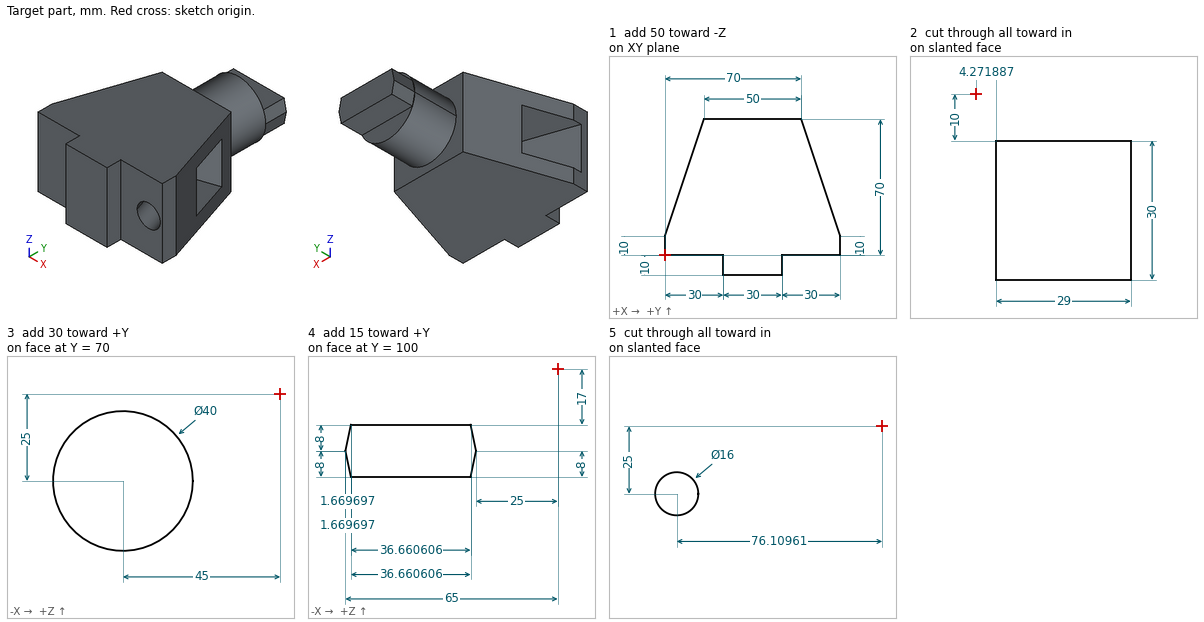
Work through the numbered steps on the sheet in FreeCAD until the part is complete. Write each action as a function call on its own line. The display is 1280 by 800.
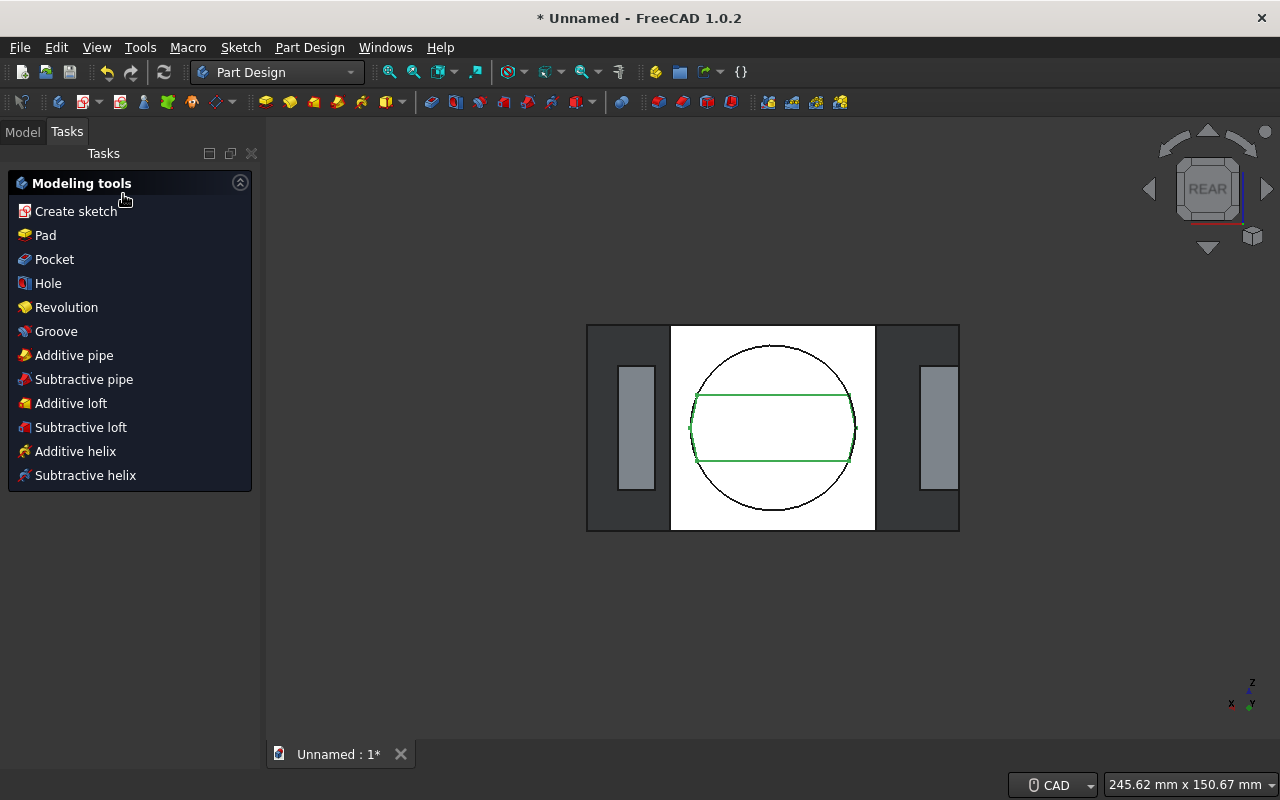
click(266, 102)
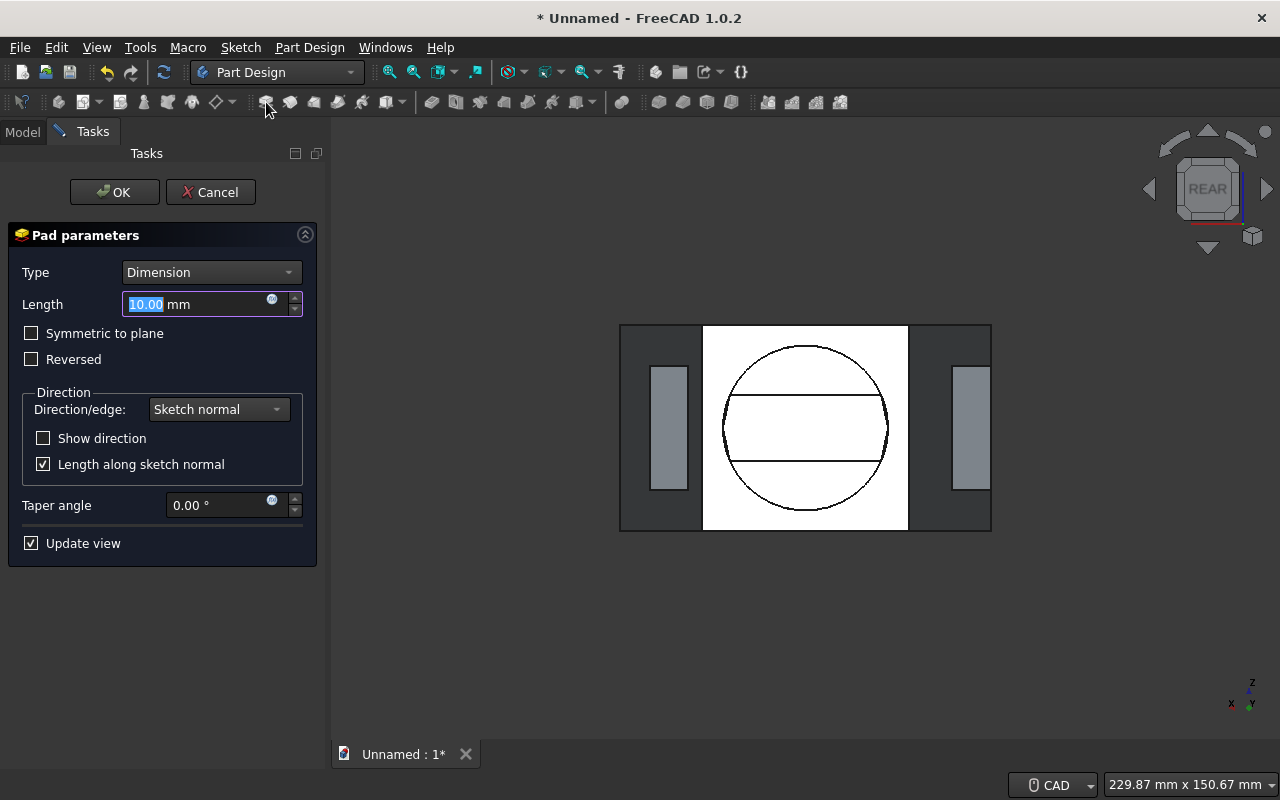
text(15)
key(Tab)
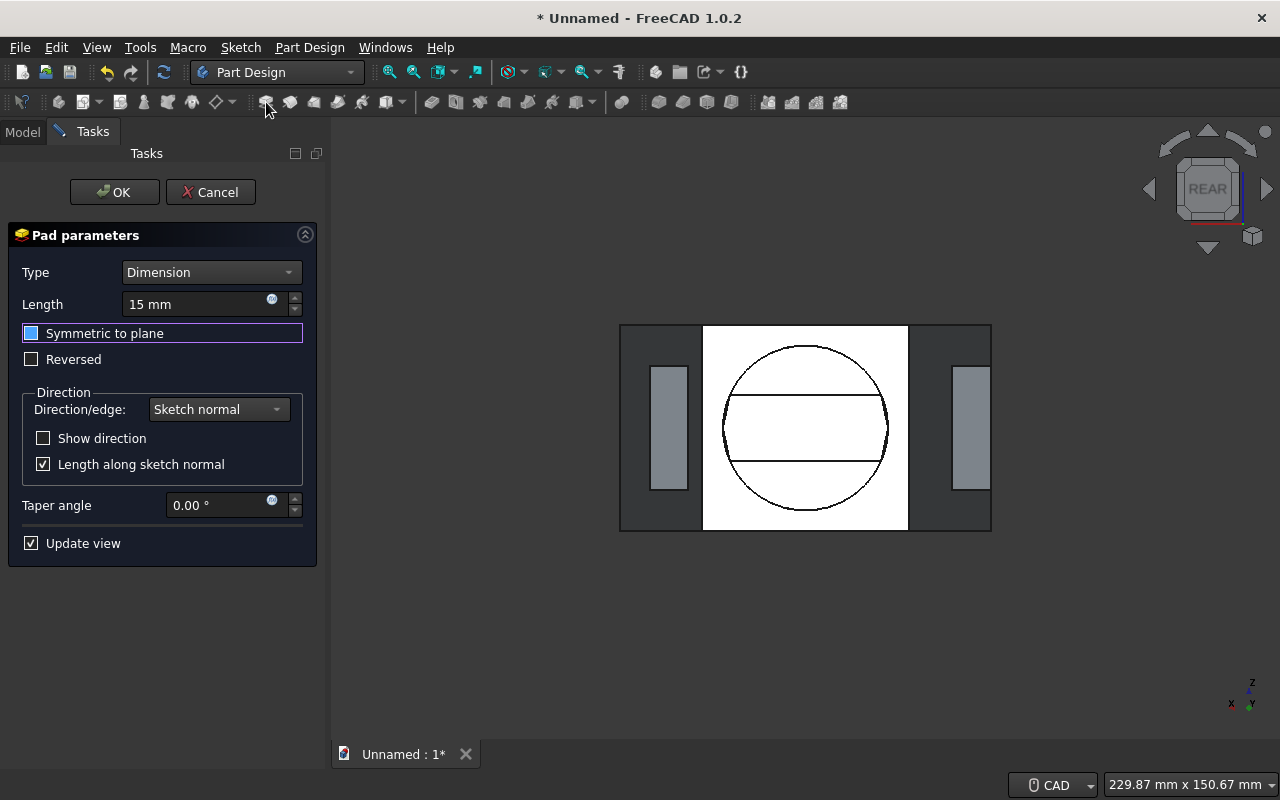
click(115, 192)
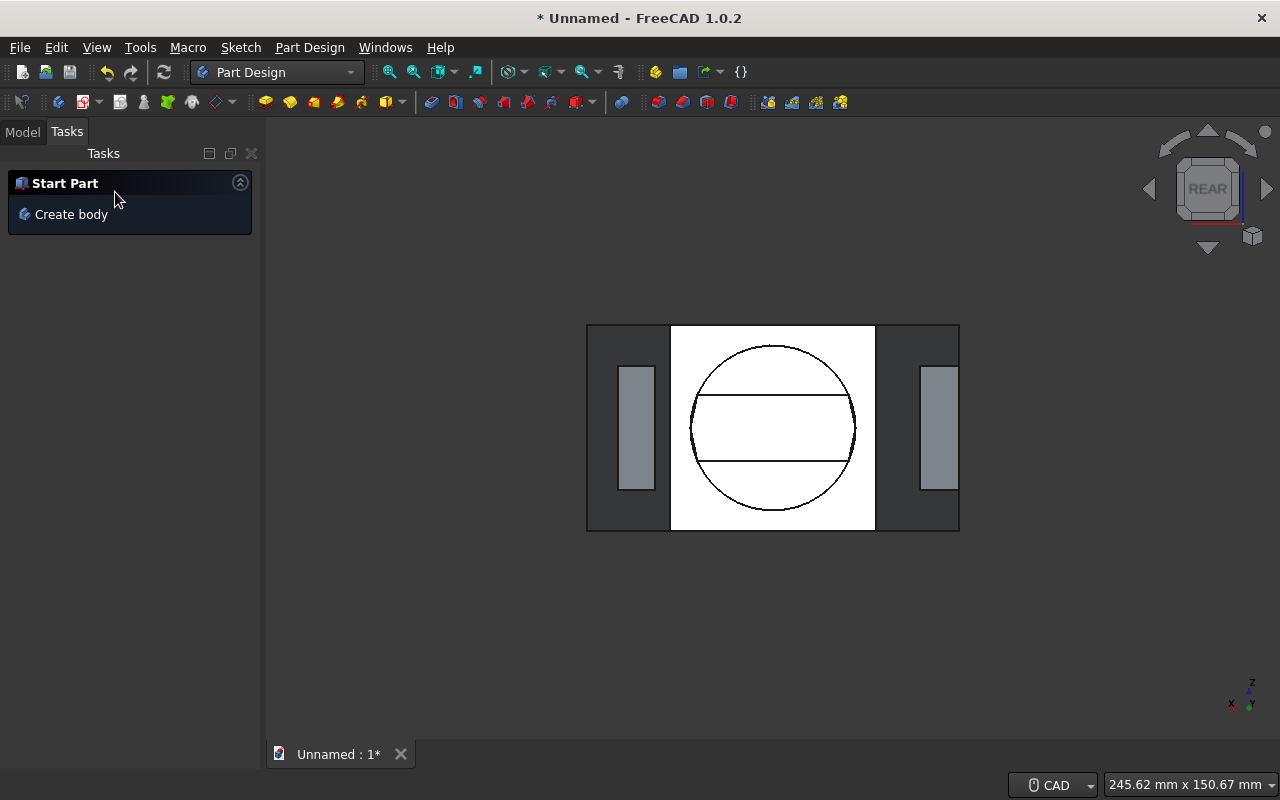
key(v)
key(f)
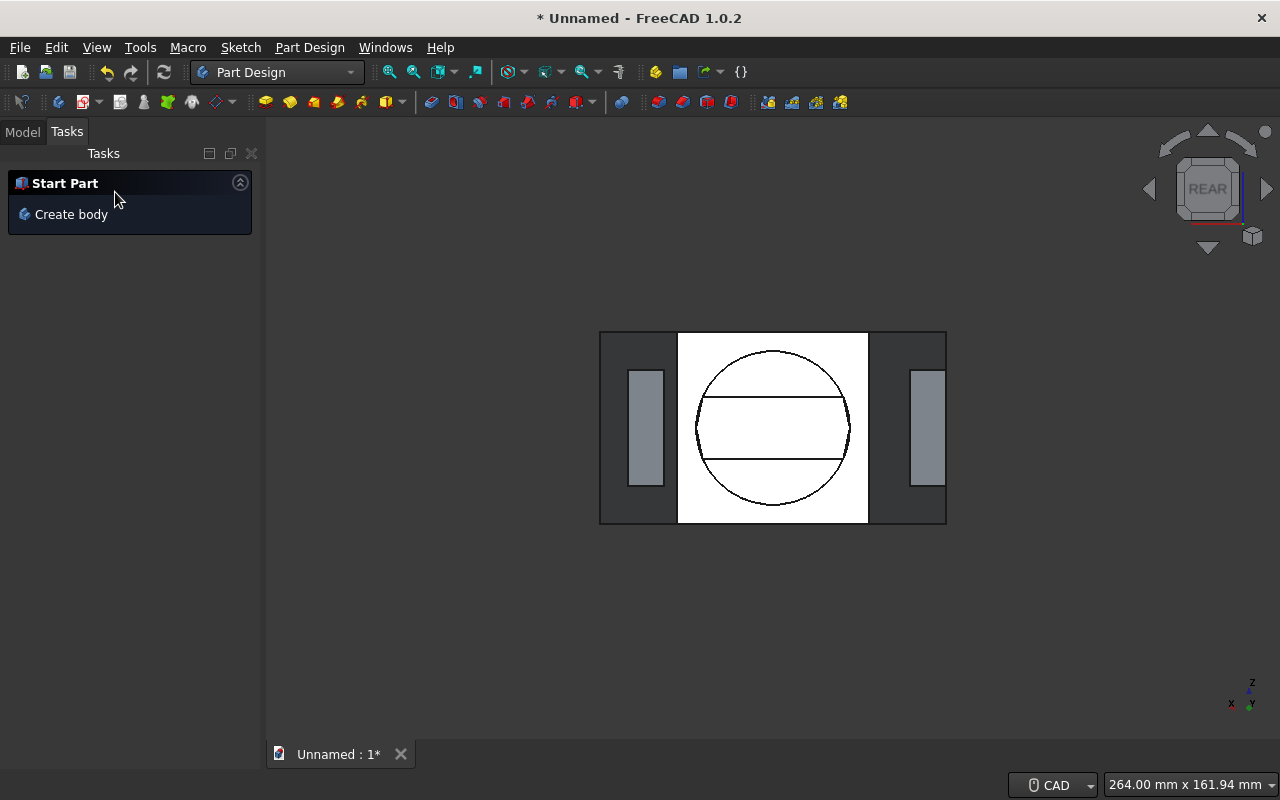
key(6)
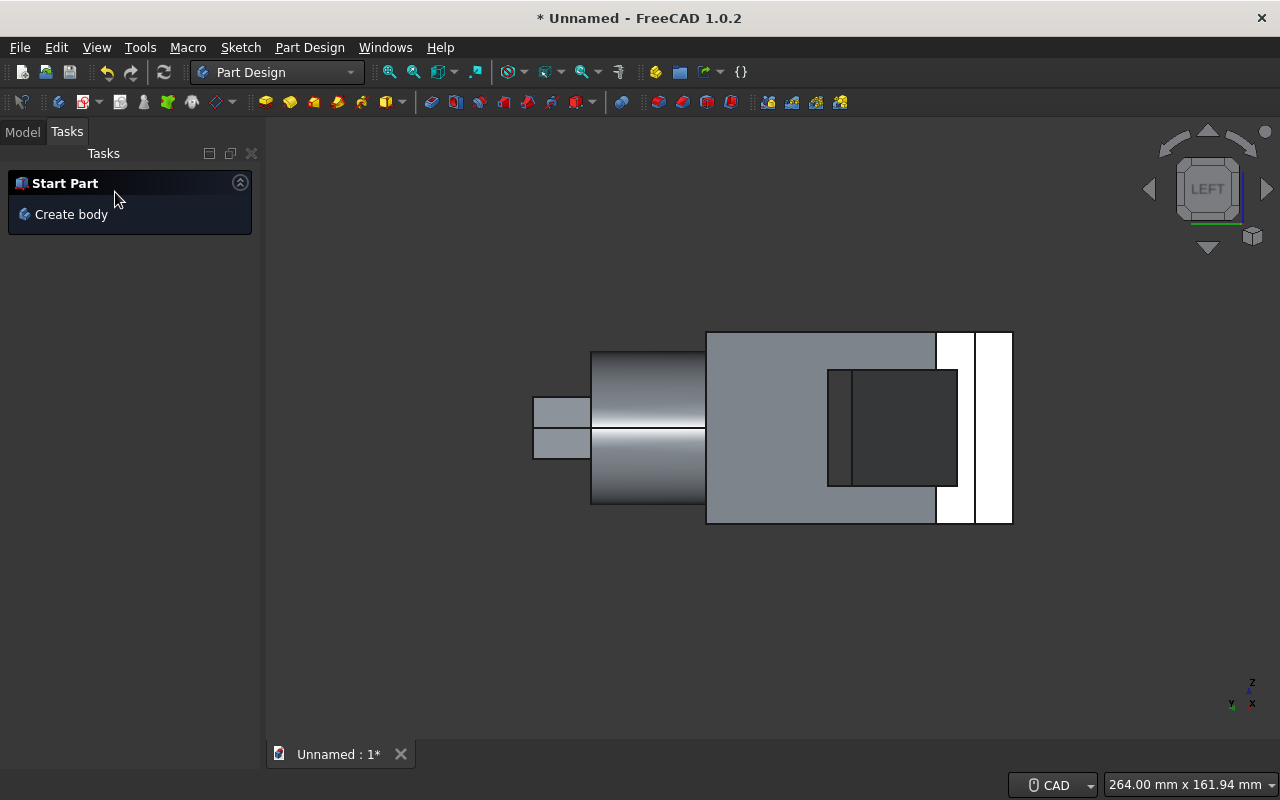
click(935, 427)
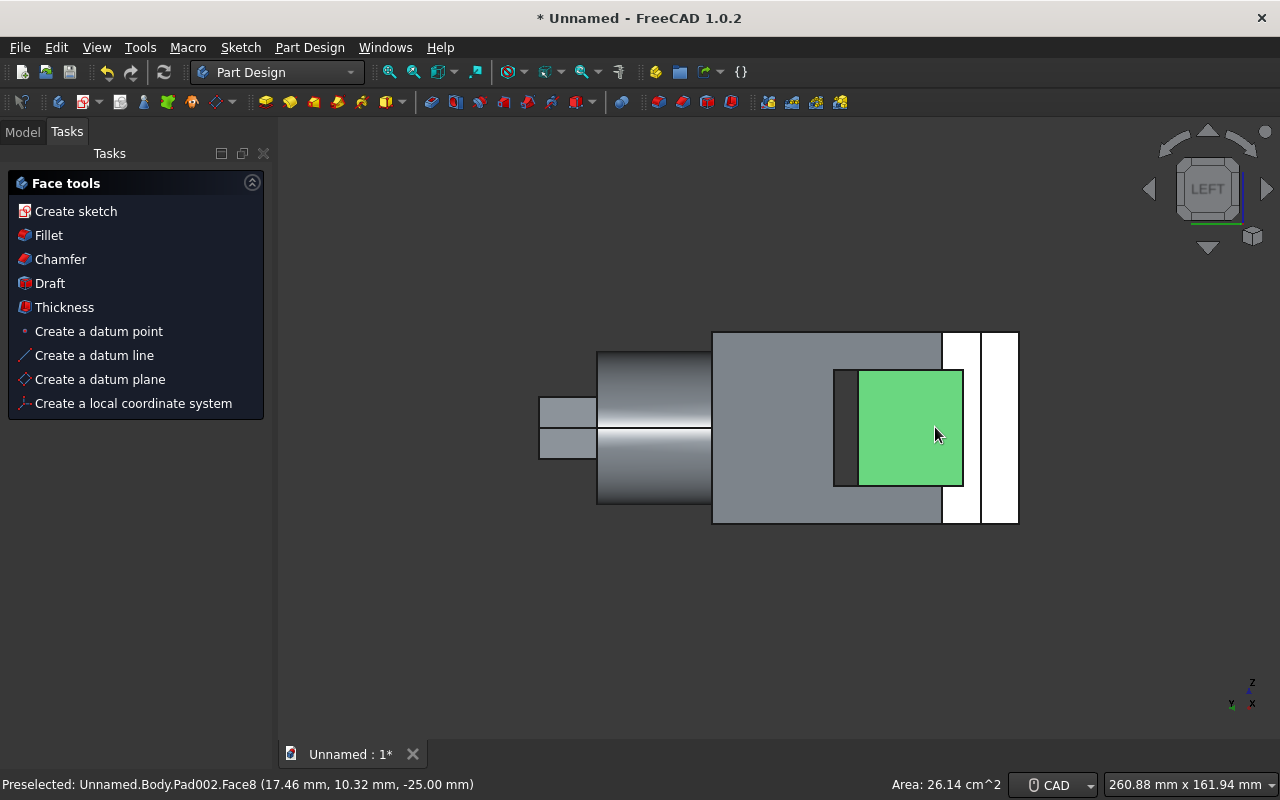
click(84, 102)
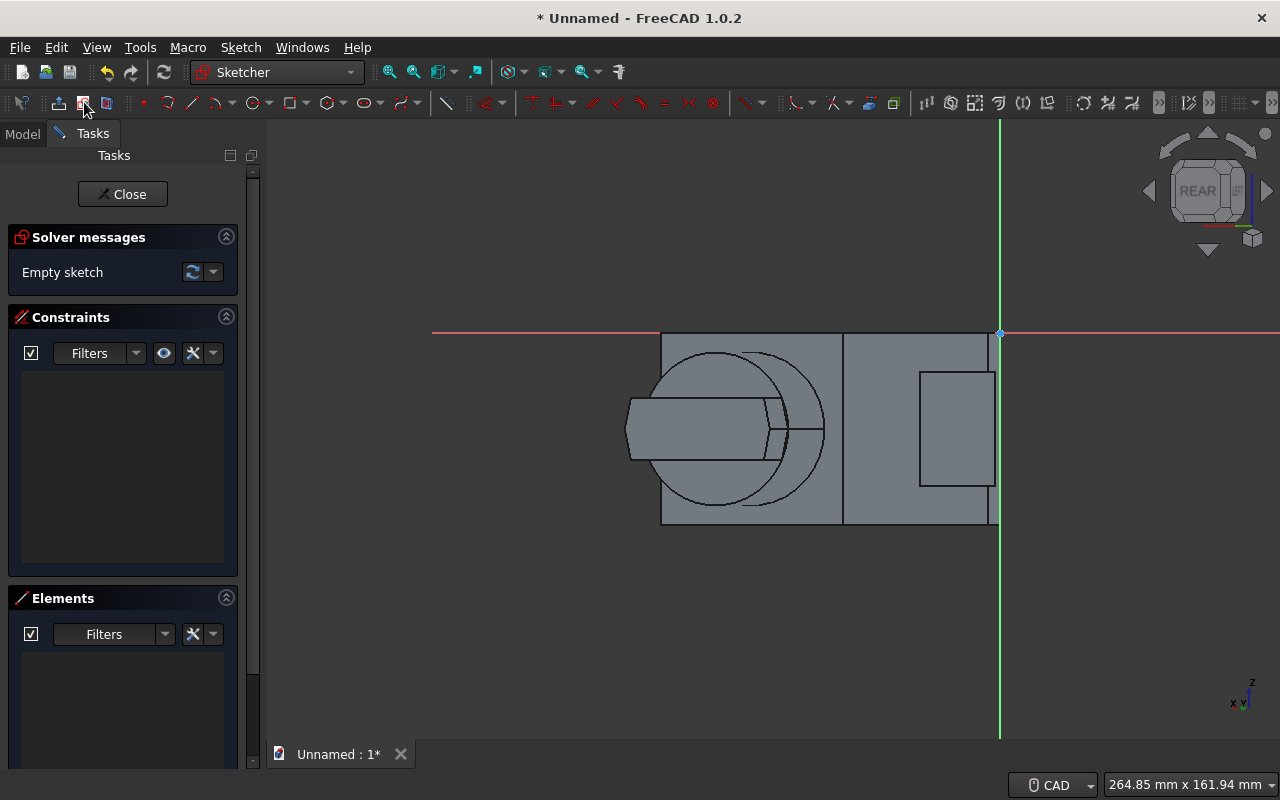
scroll(709, 429, up, 9)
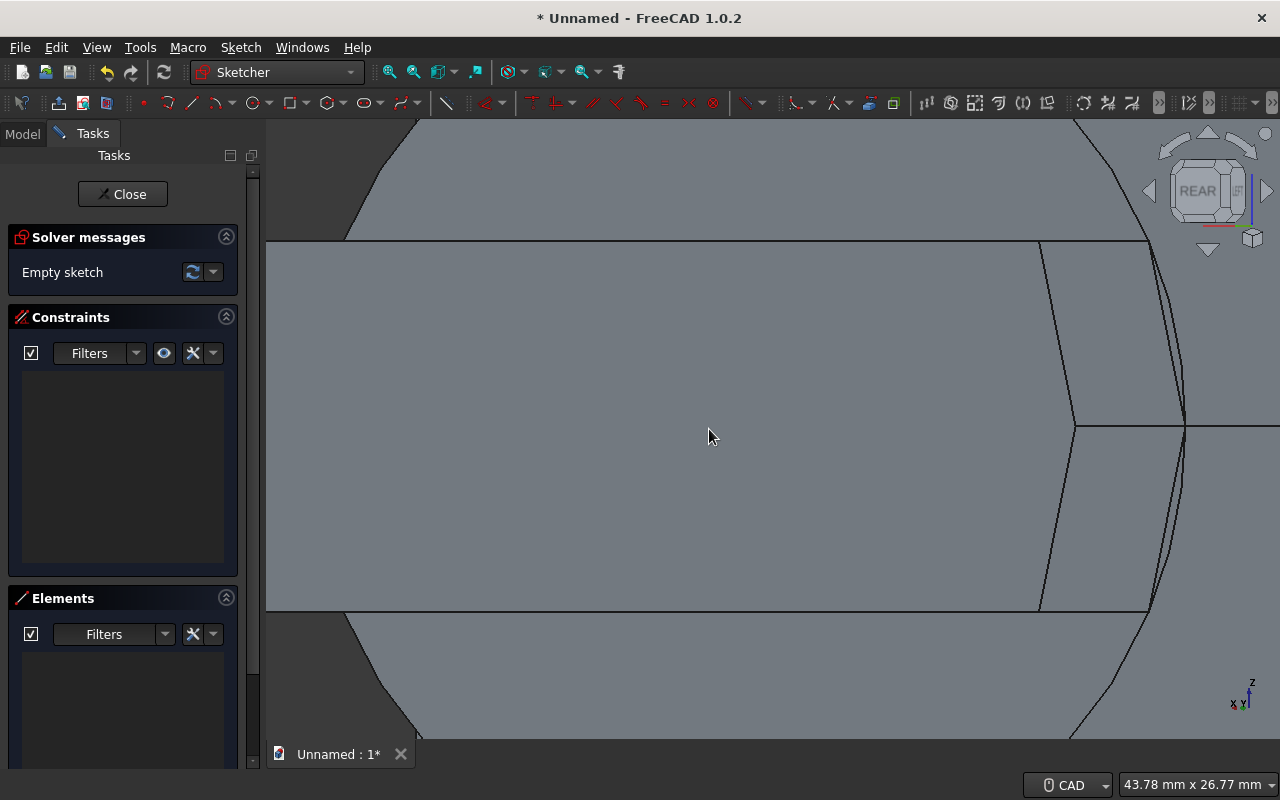
key(g)
key(c)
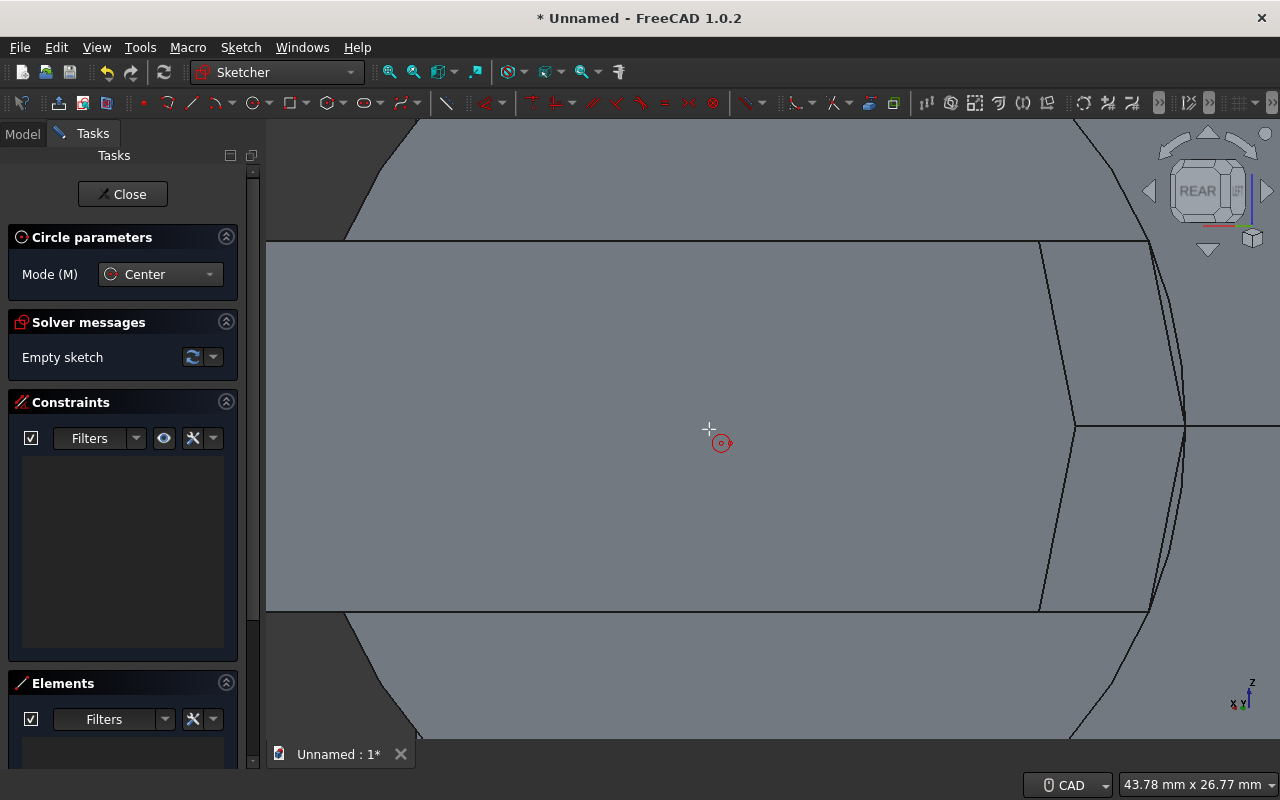
click(704, 426)
move(835, 295)